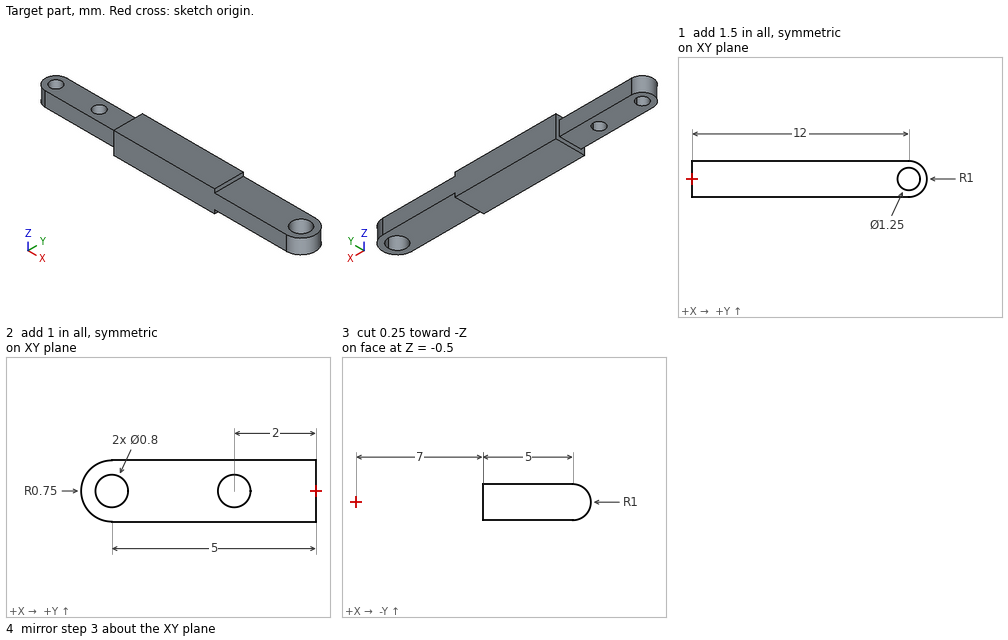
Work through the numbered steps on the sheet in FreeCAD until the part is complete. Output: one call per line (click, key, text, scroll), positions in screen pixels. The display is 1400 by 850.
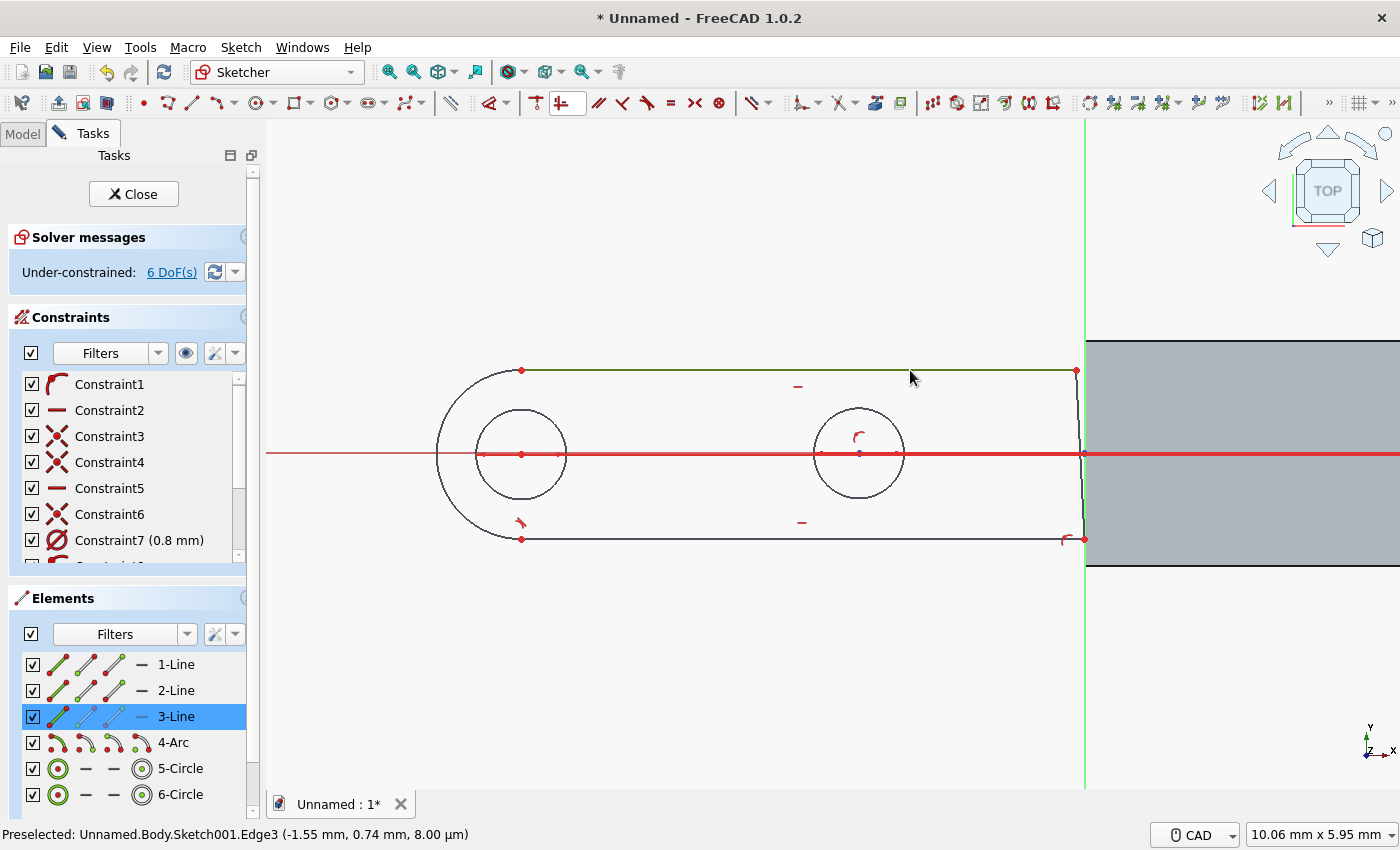
click(453, 405)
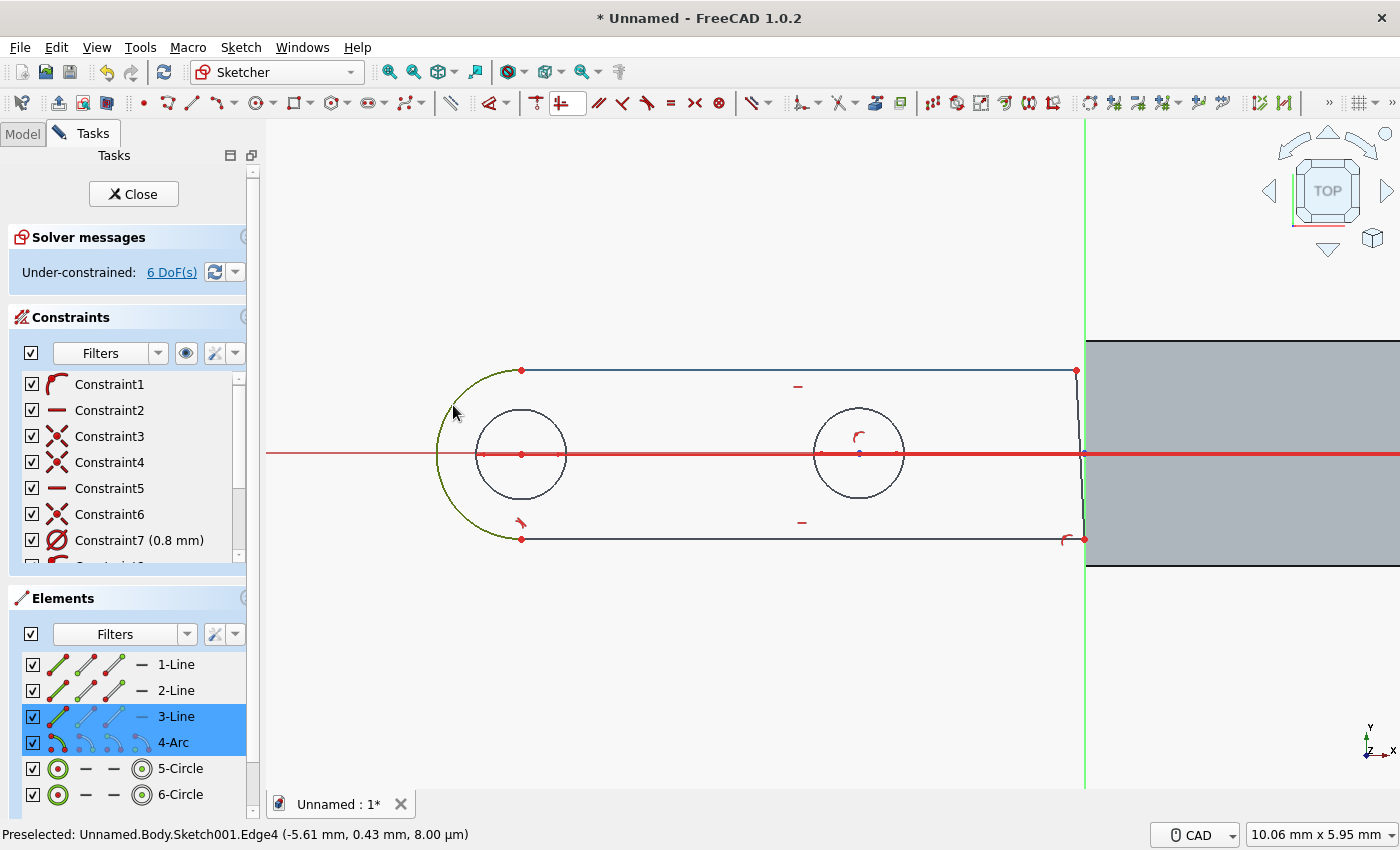
click(648, 104)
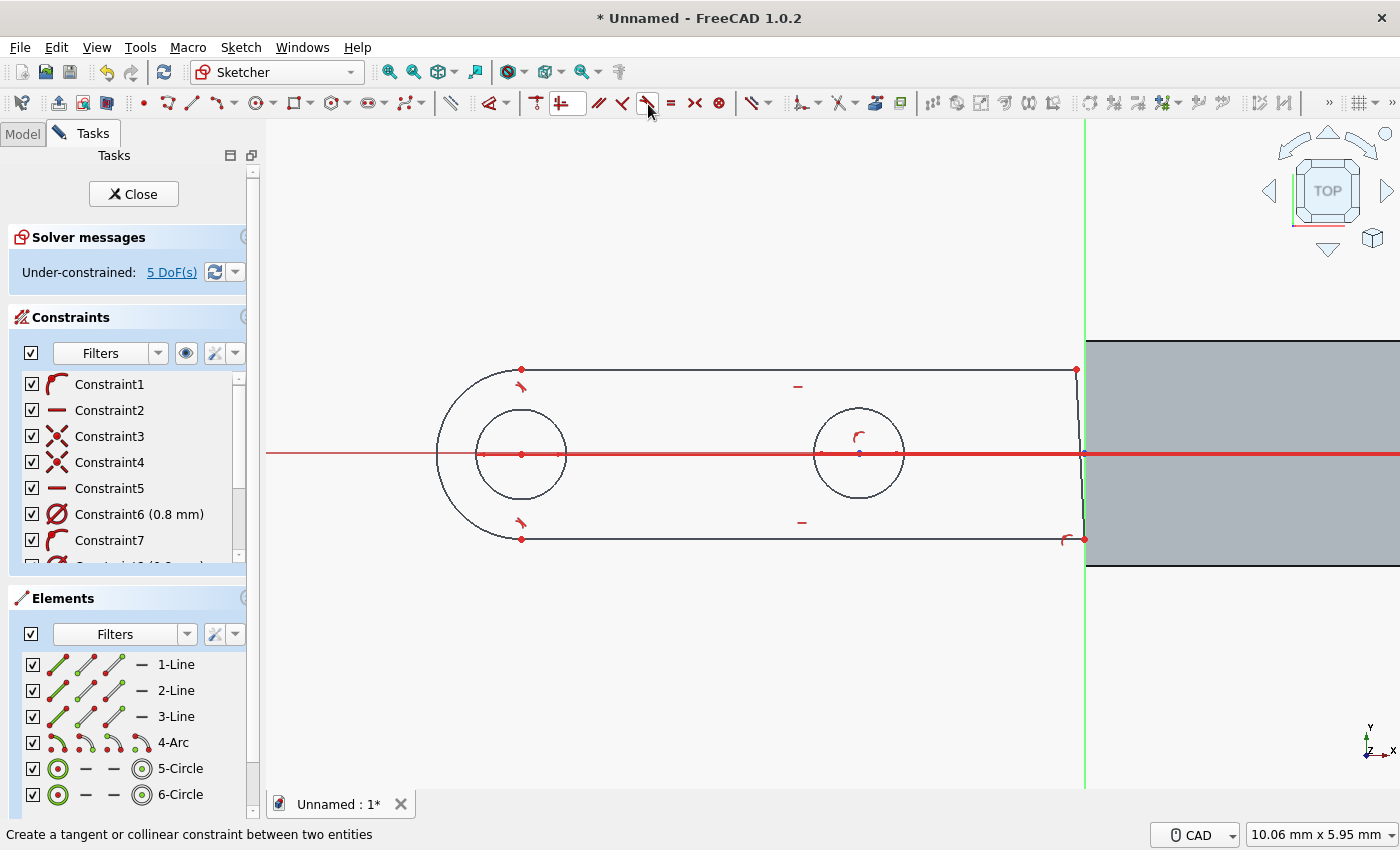
click(1082, 488)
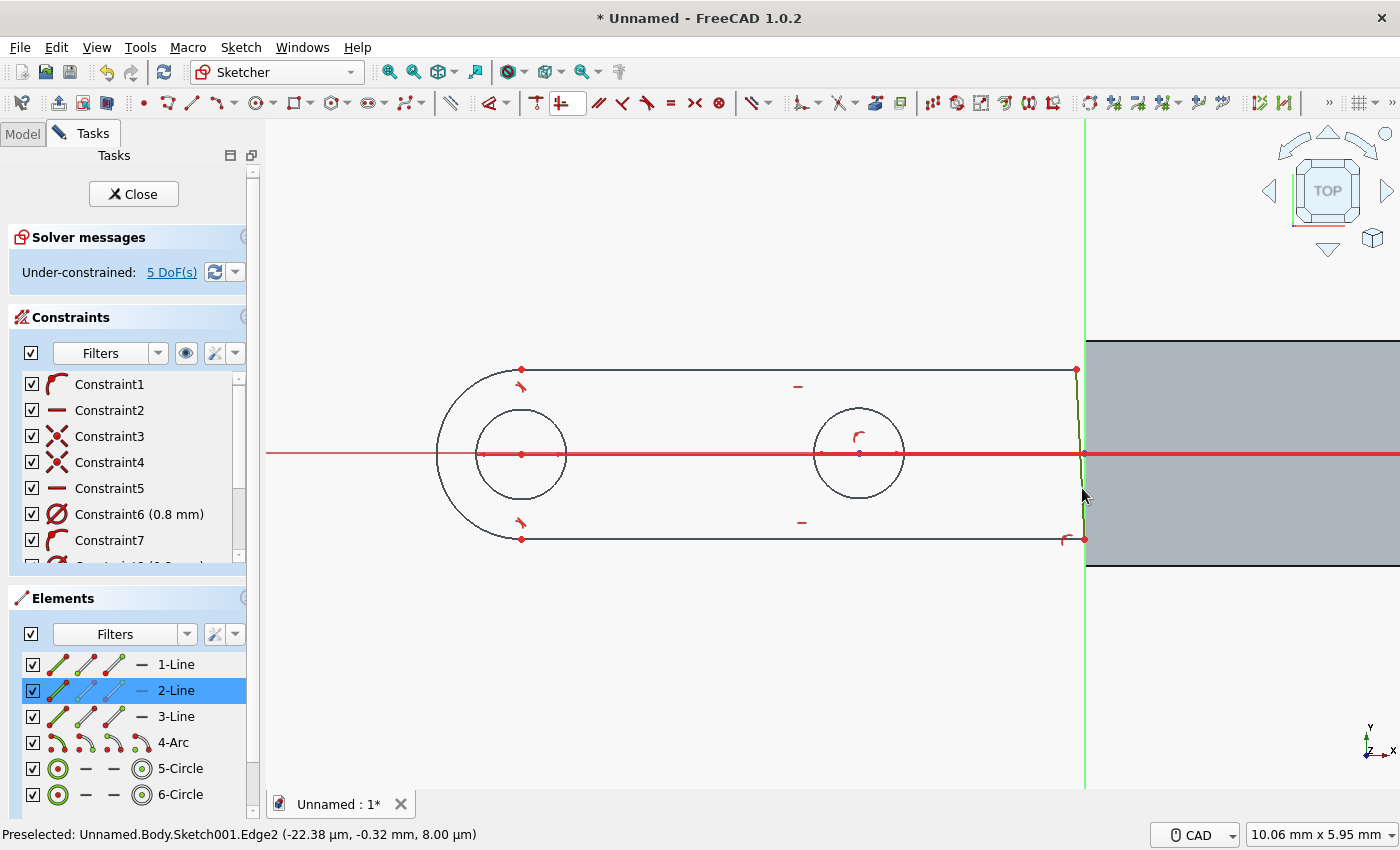
click(580, 104)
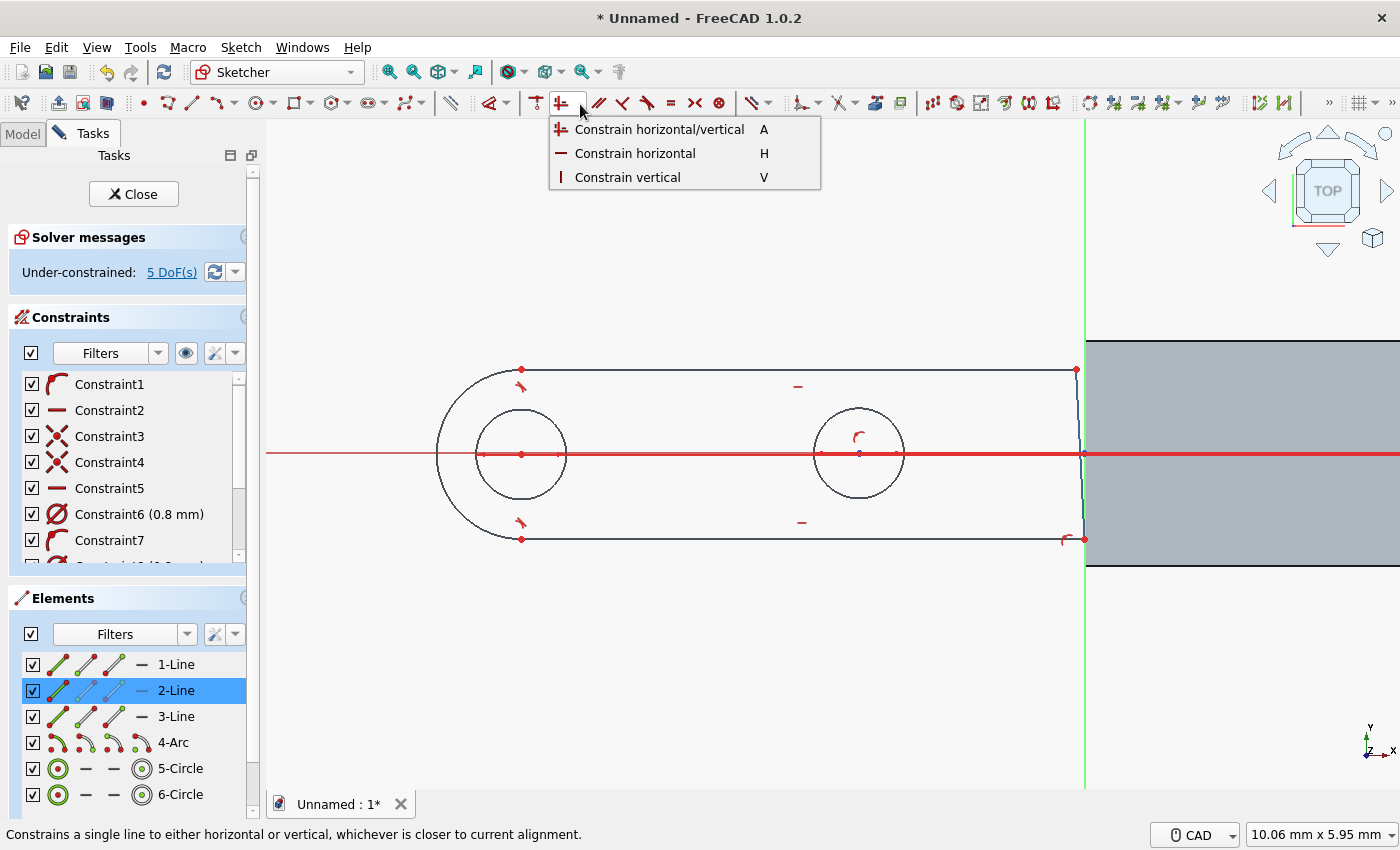
click(685, 177)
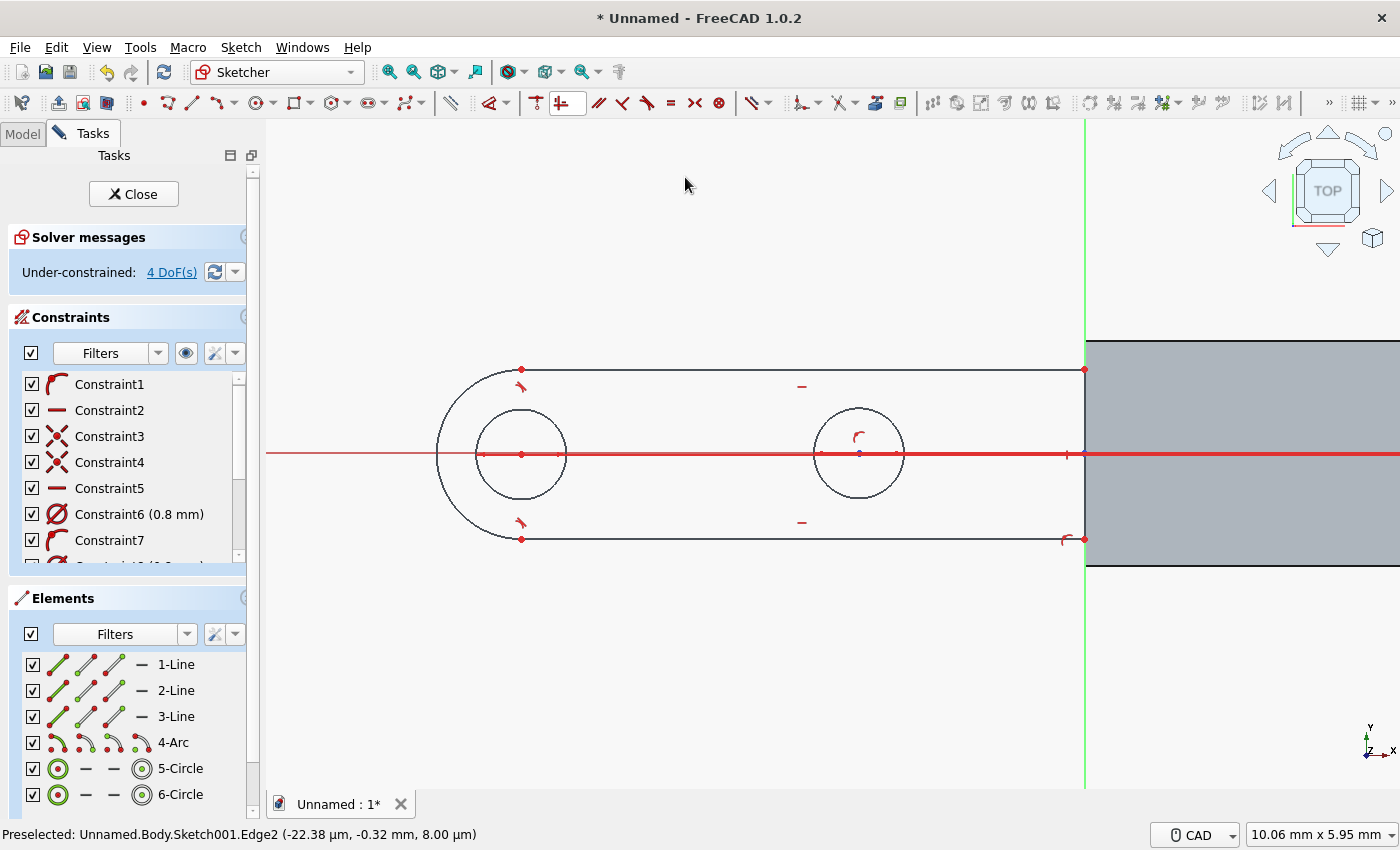
click(521, 455)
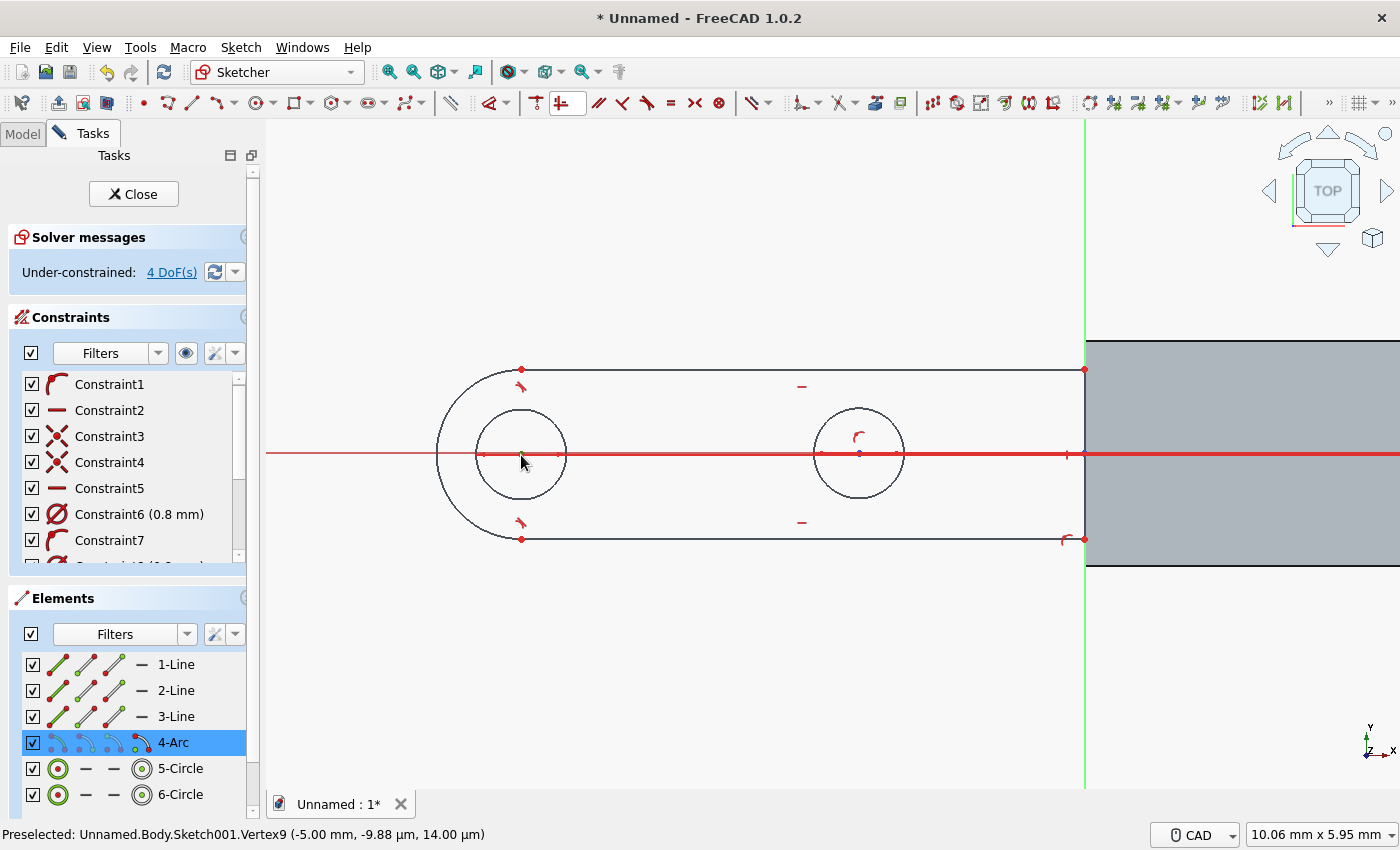
click(361, 453)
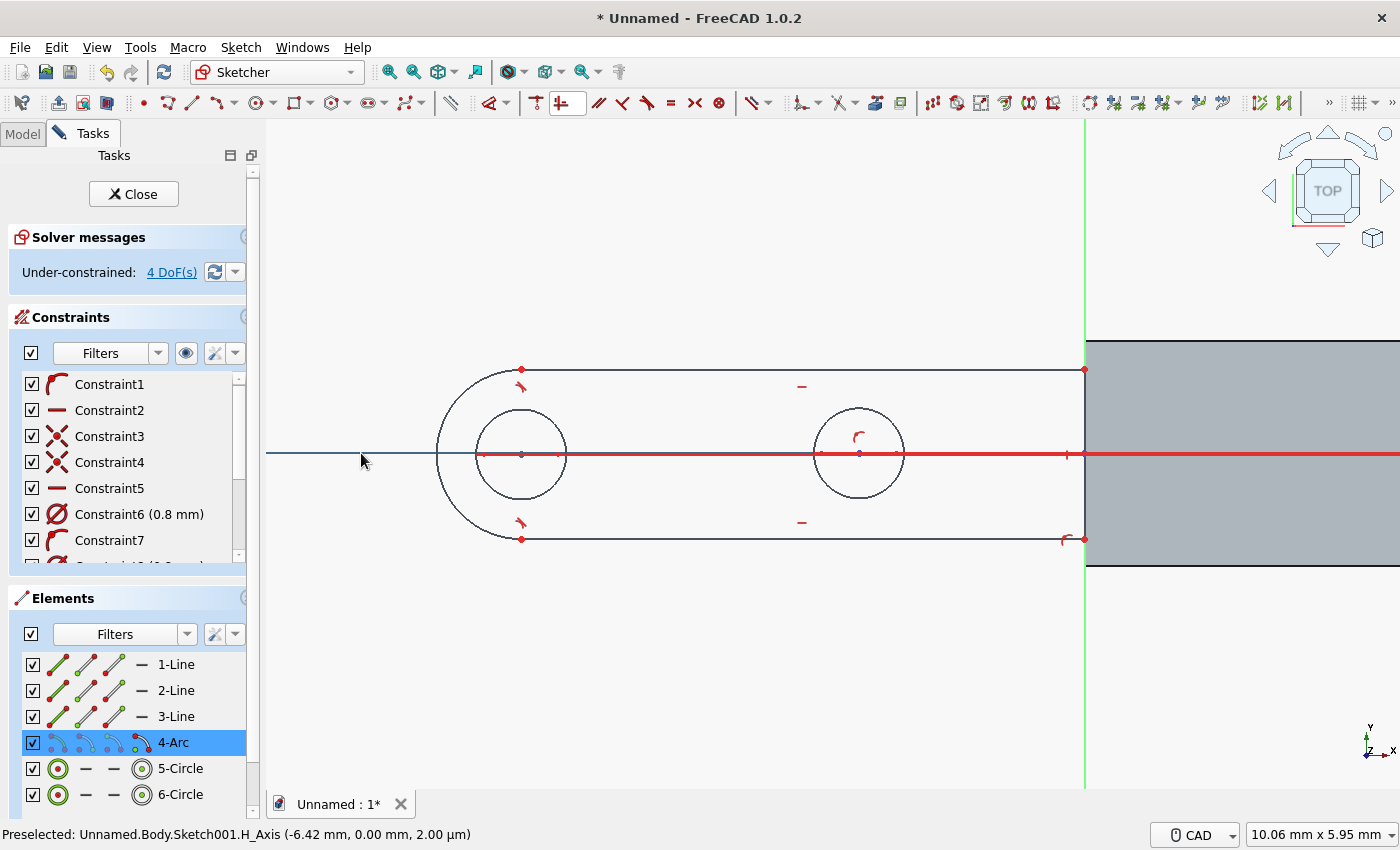
click(536, 104)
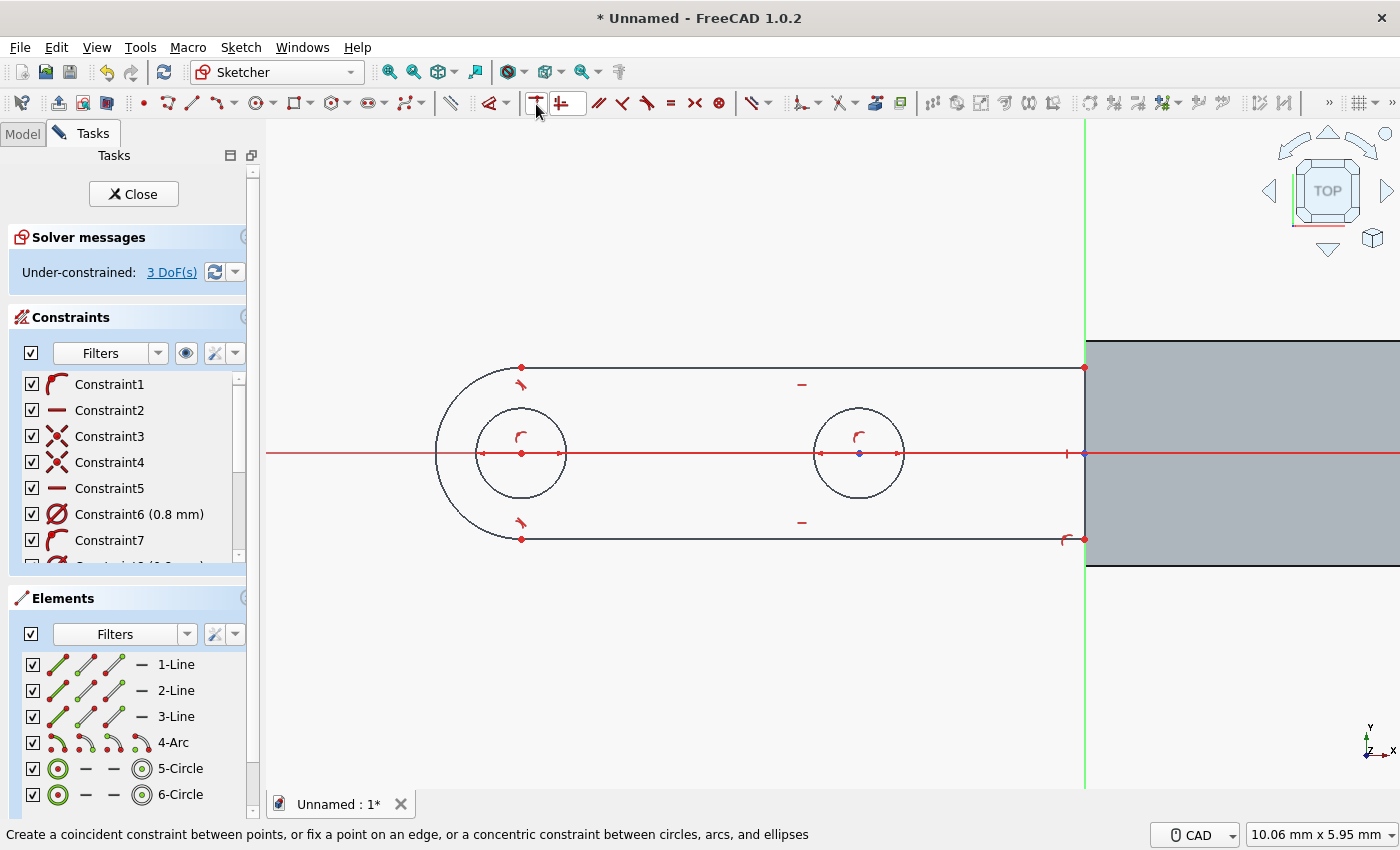
click(490, 104)